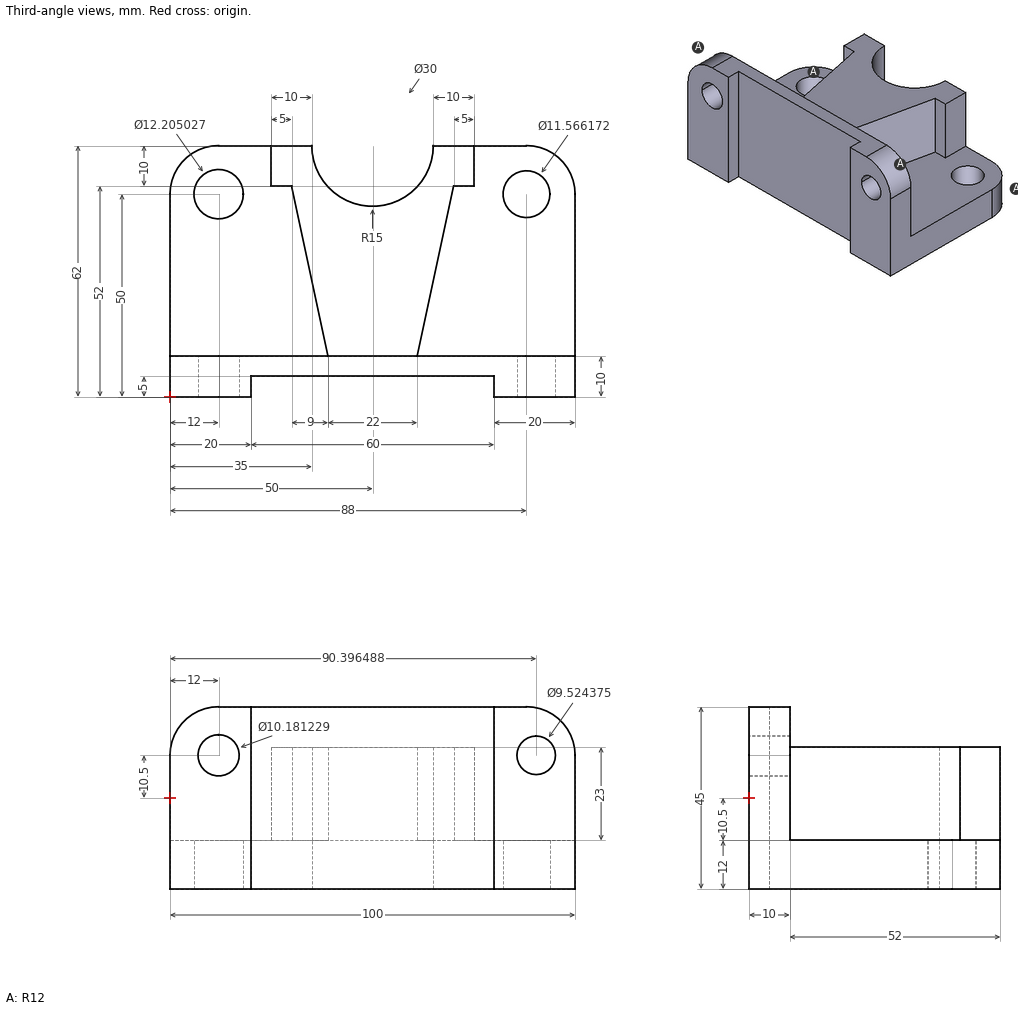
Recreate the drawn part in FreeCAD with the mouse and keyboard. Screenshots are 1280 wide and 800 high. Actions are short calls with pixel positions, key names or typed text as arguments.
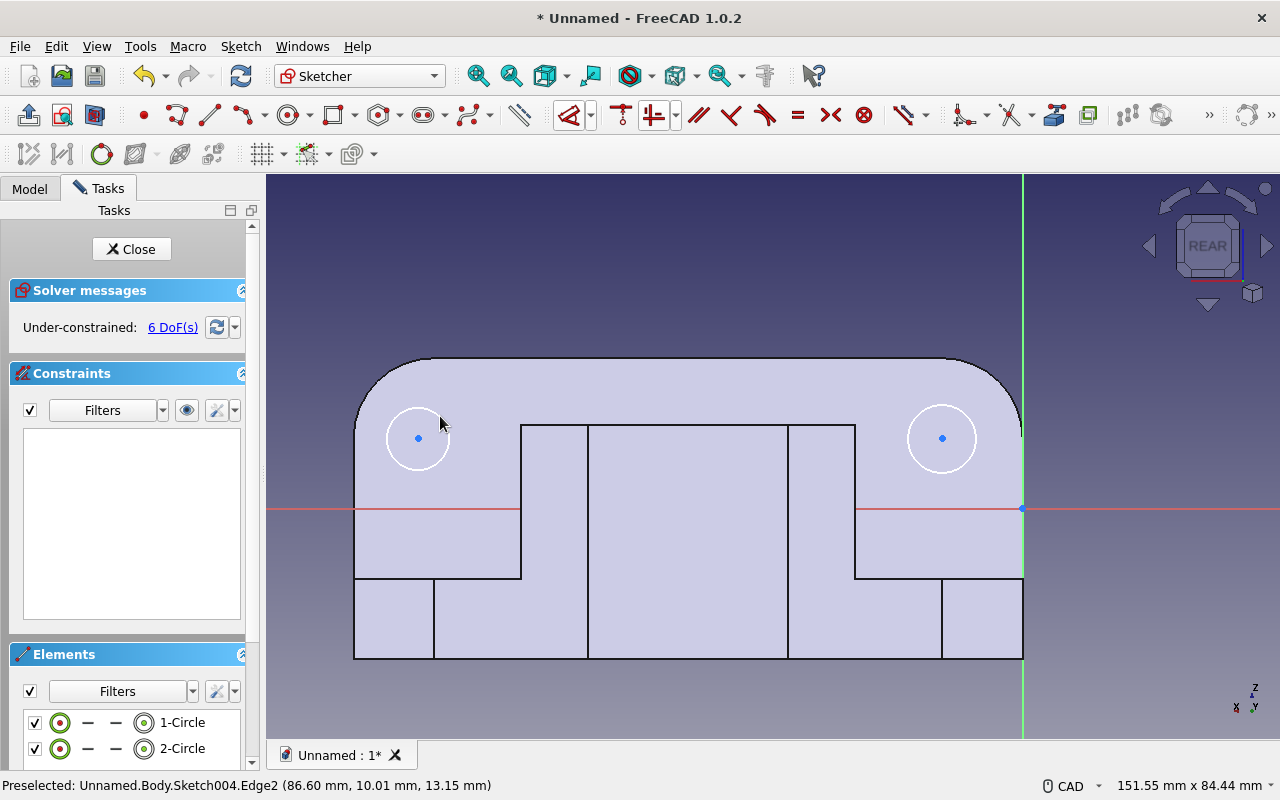
click(942, 439)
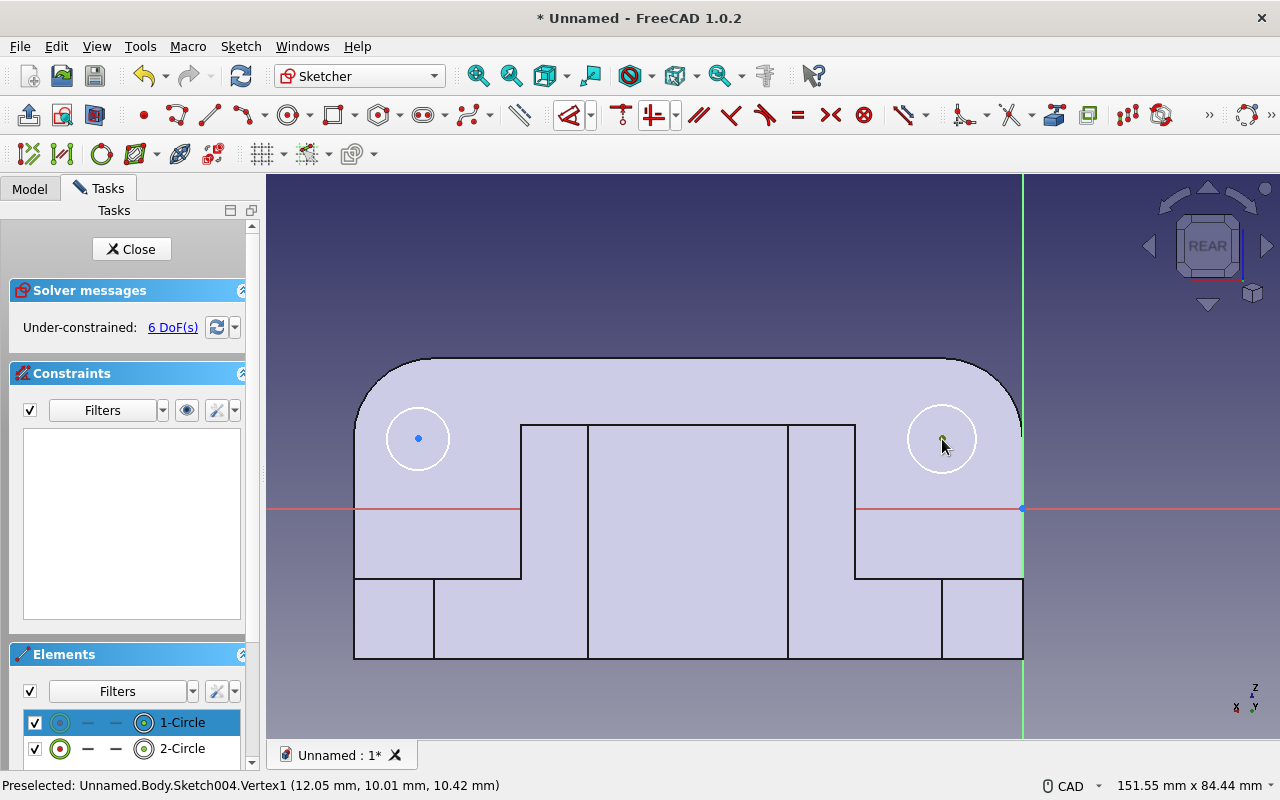
click(418, 439)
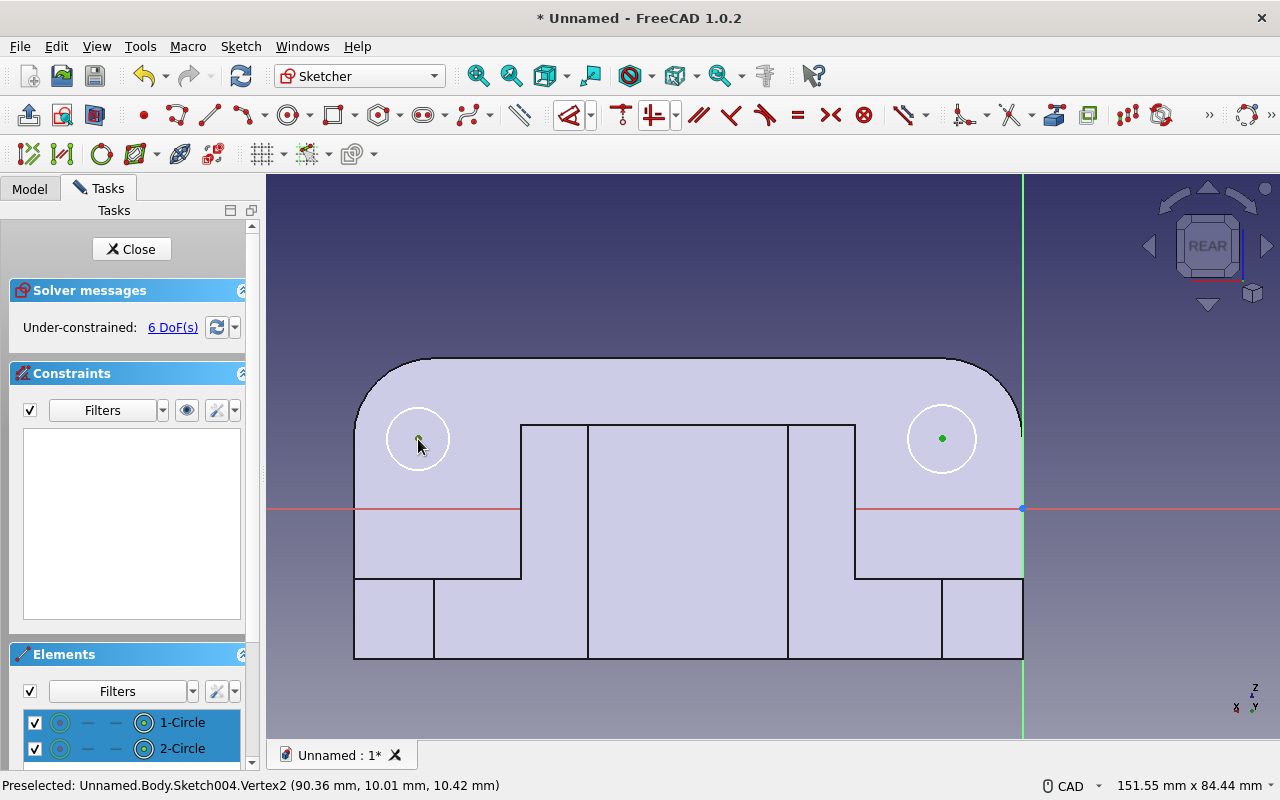
key(h)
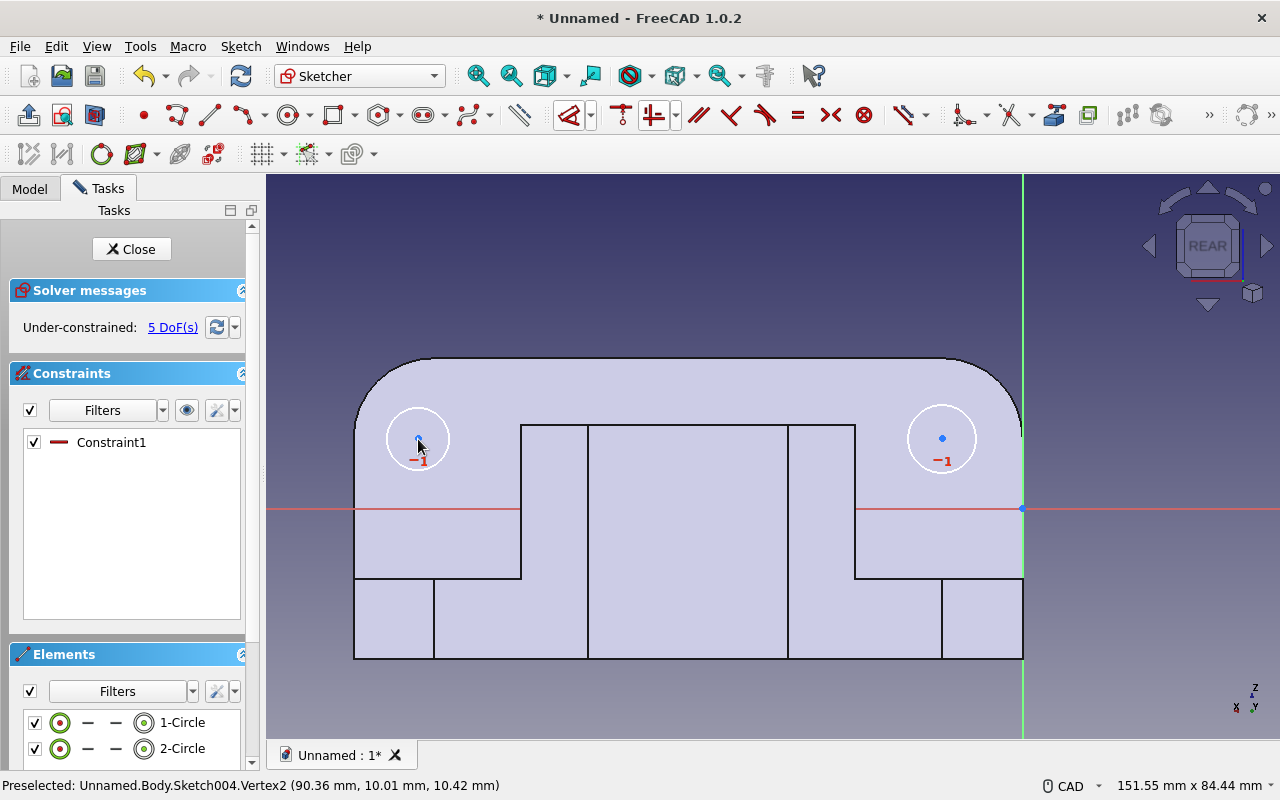
click(966, 415)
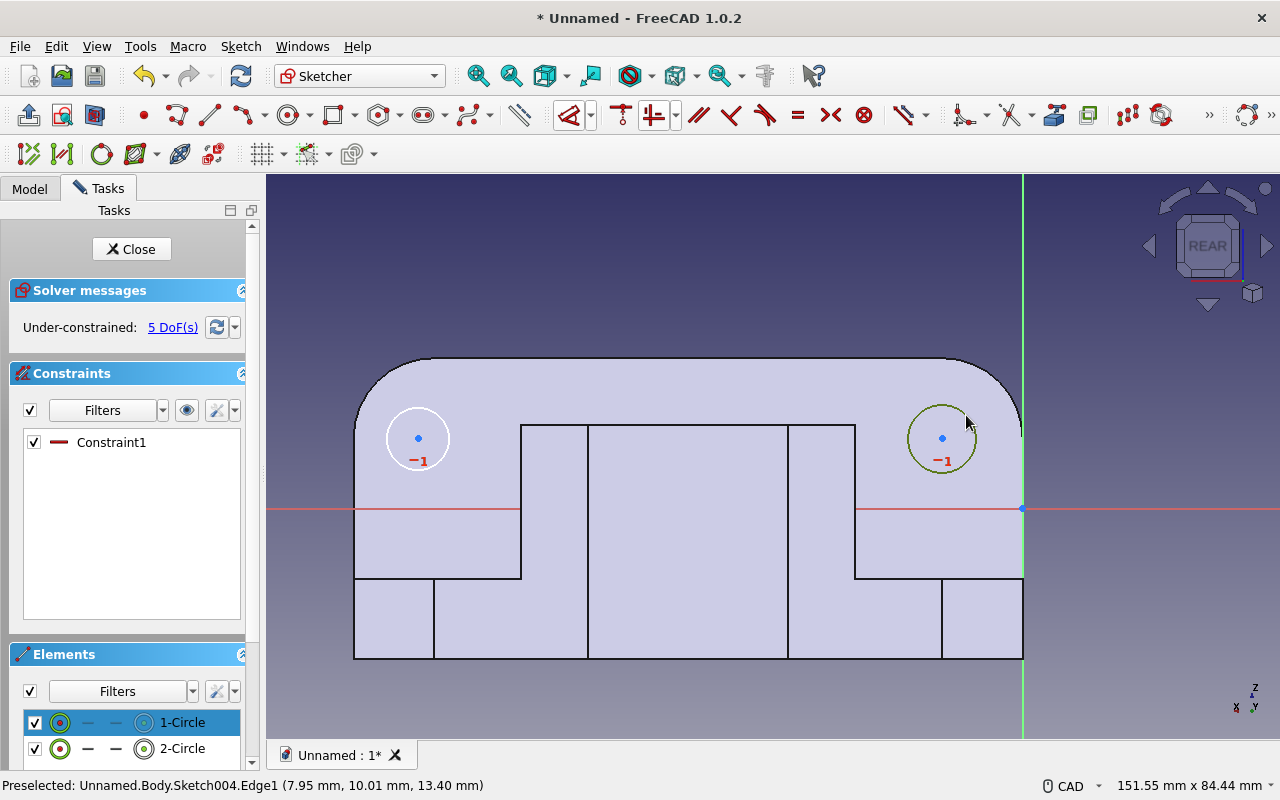
key(k)
key(o)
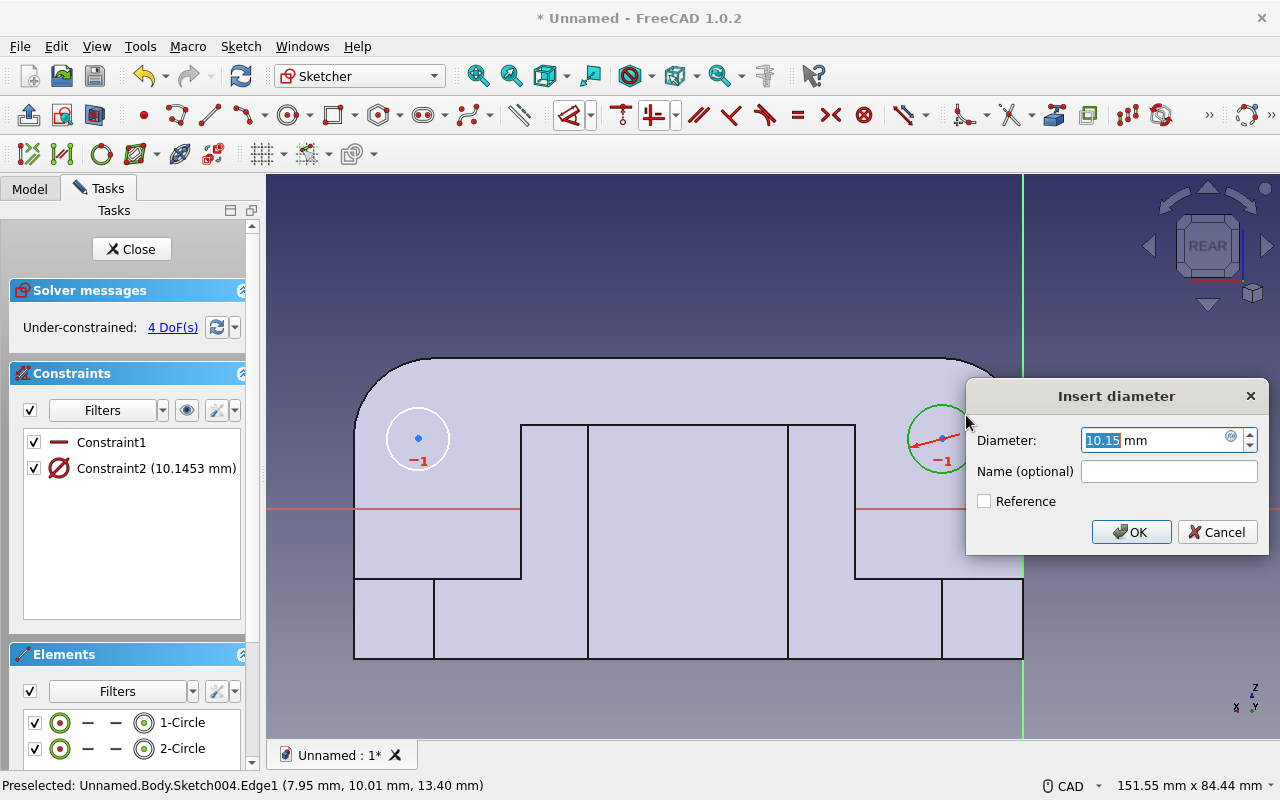
text(10.181229)
key(Return)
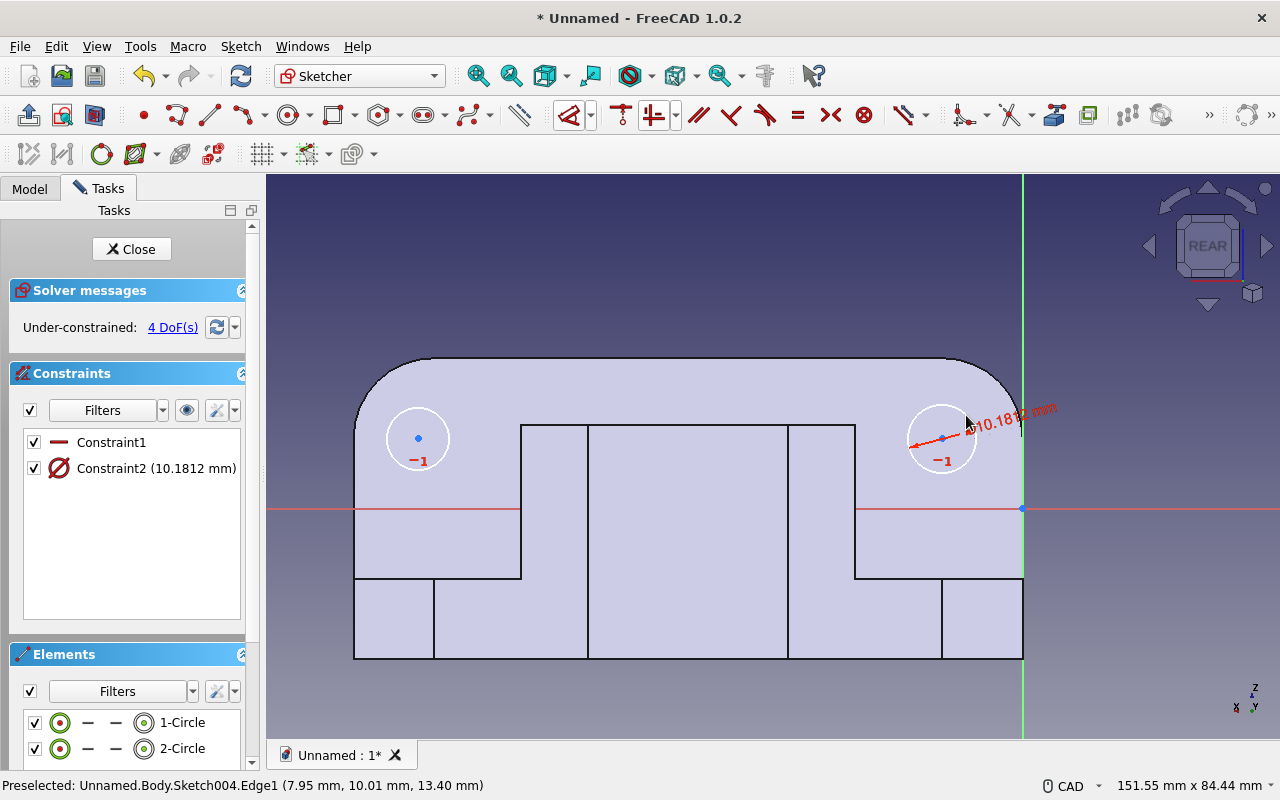
click(440, 417)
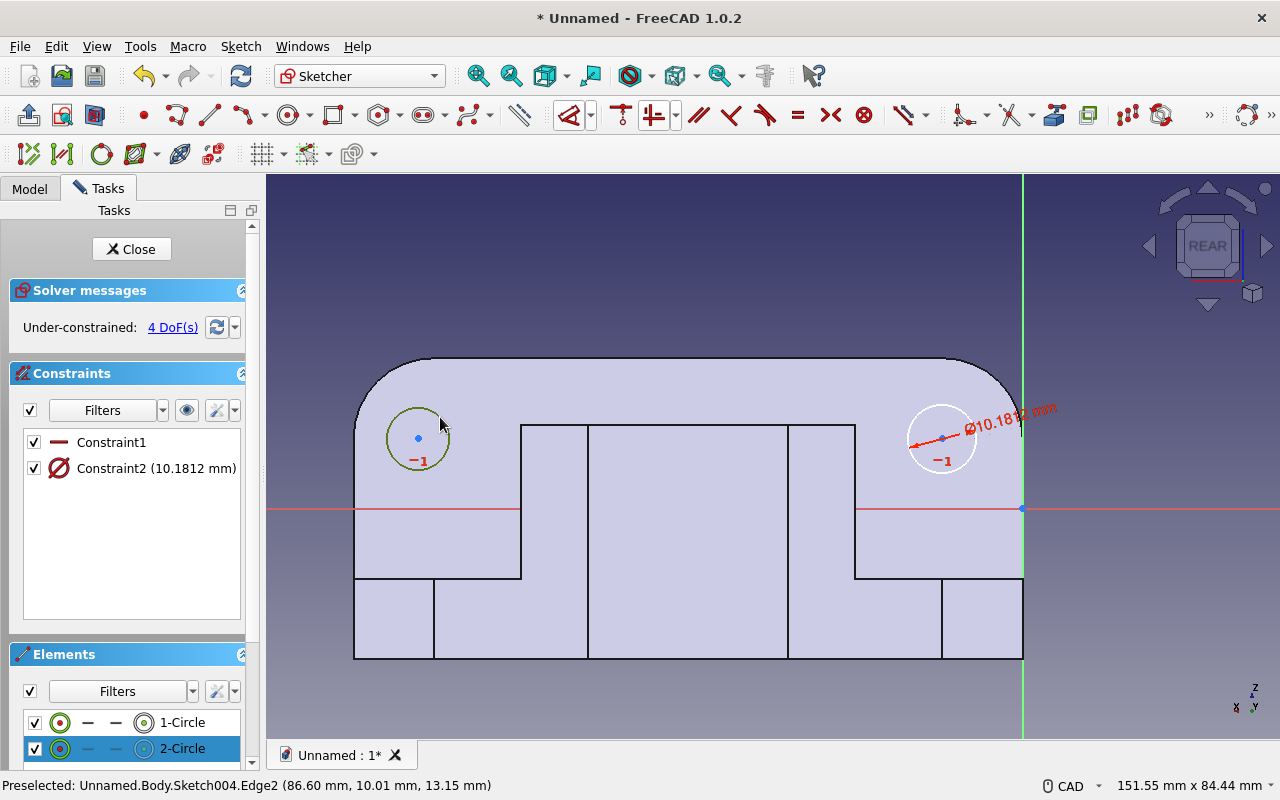
key(k)
key(o)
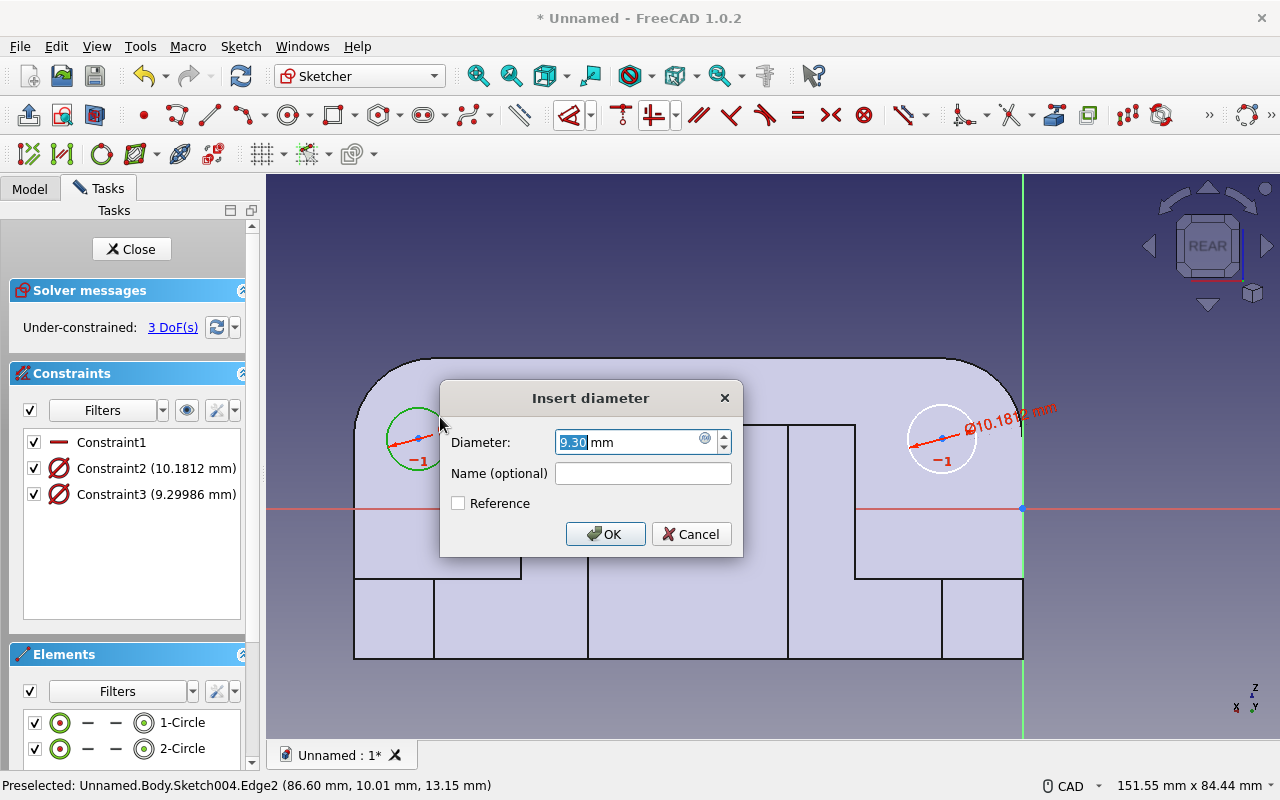
text(9.524375)
key(Return)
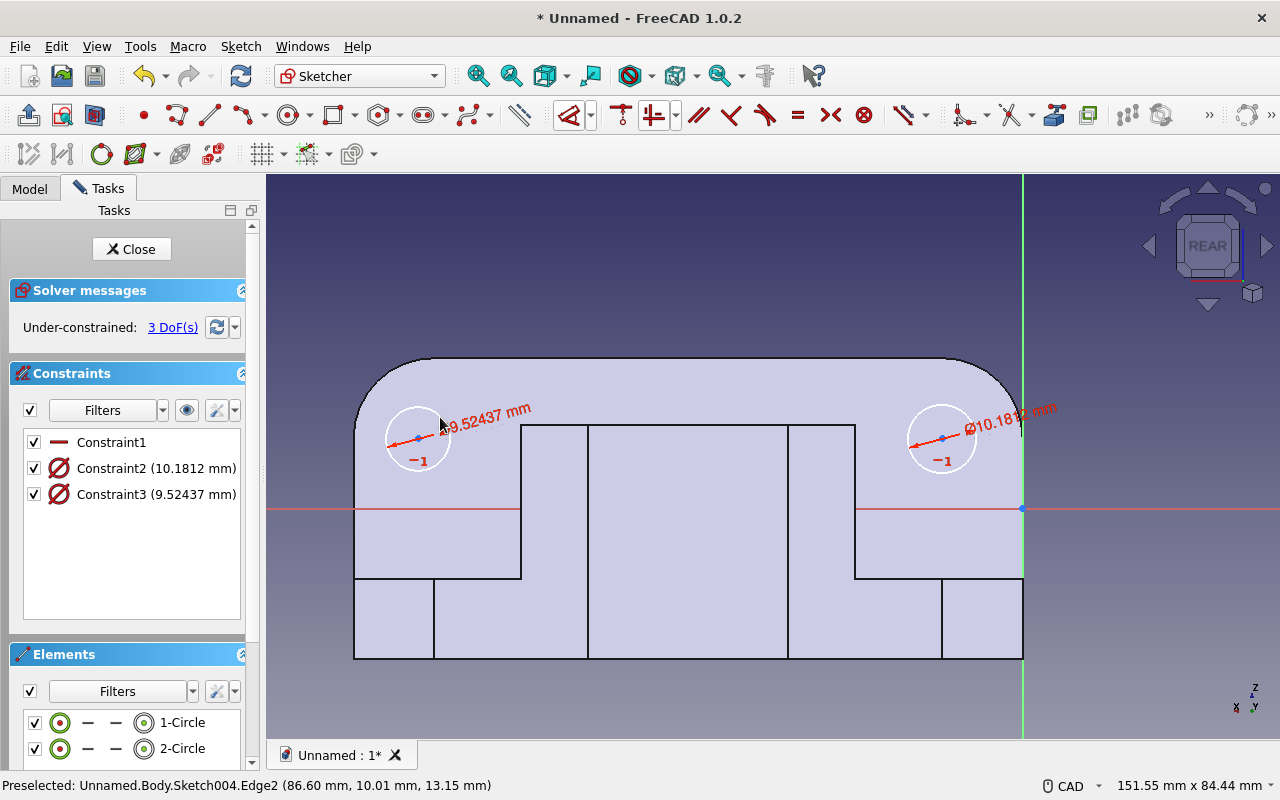
click(942, 439)